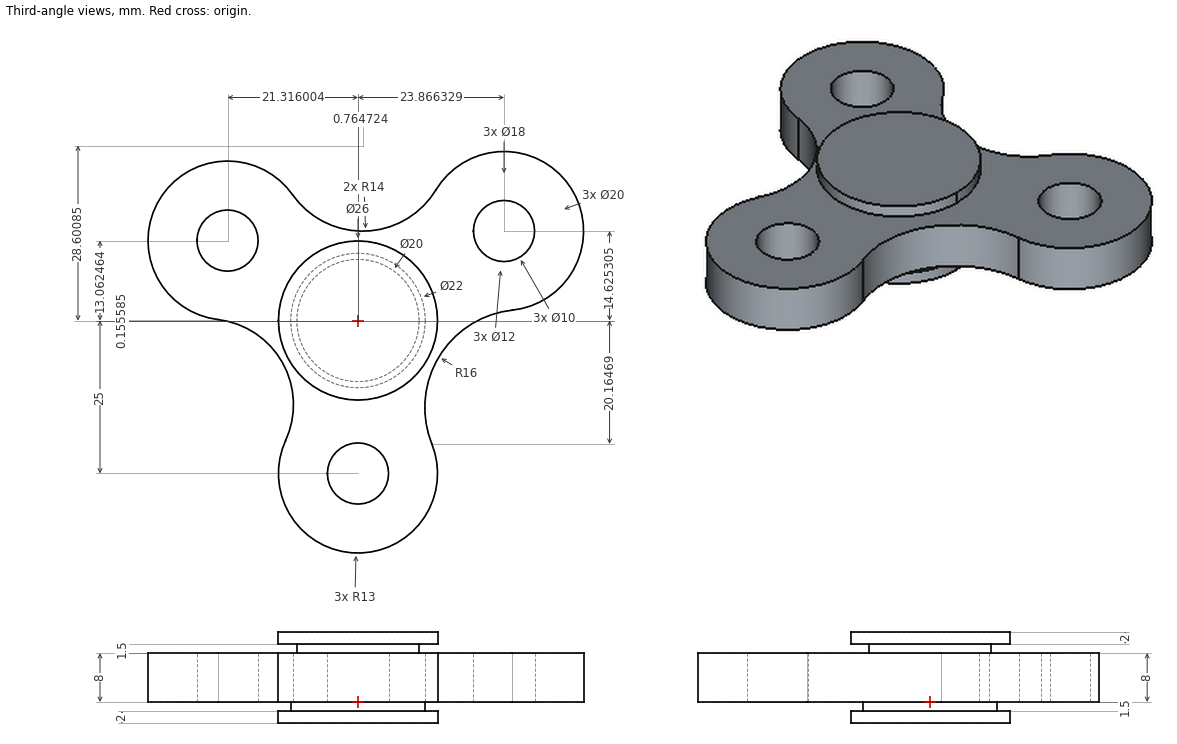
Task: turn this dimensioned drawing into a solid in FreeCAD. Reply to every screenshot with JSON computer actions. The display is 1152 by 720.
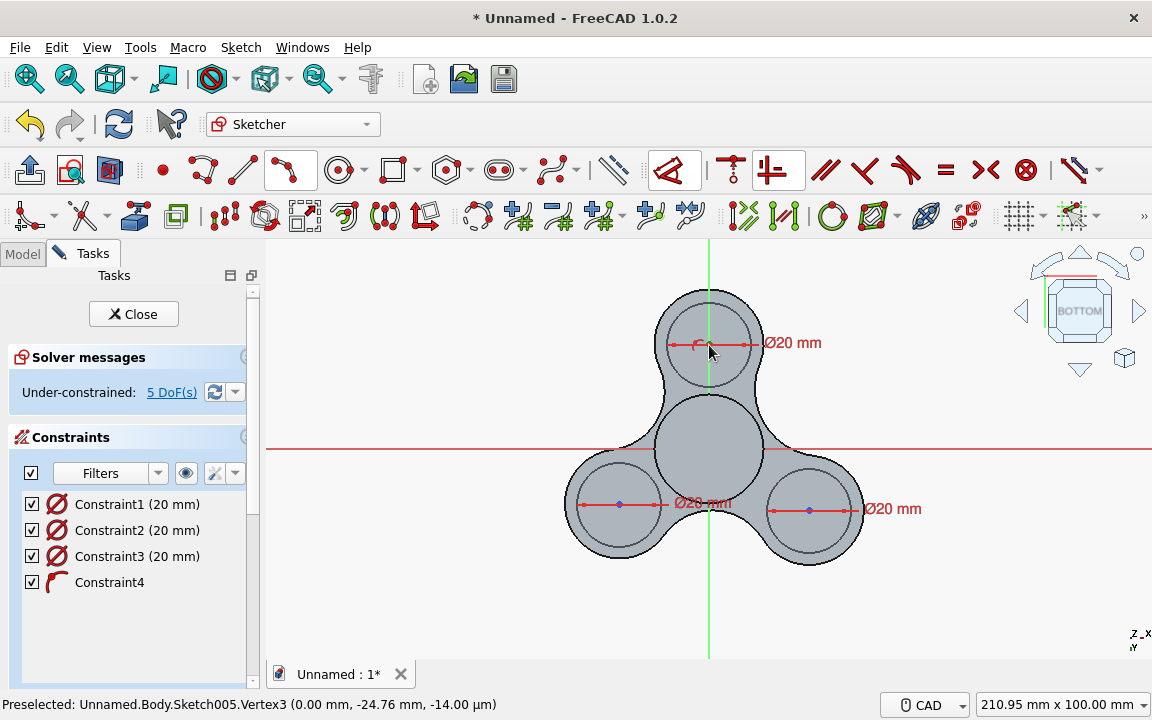
{"action": "left_click", "coordinate": [696, 170]}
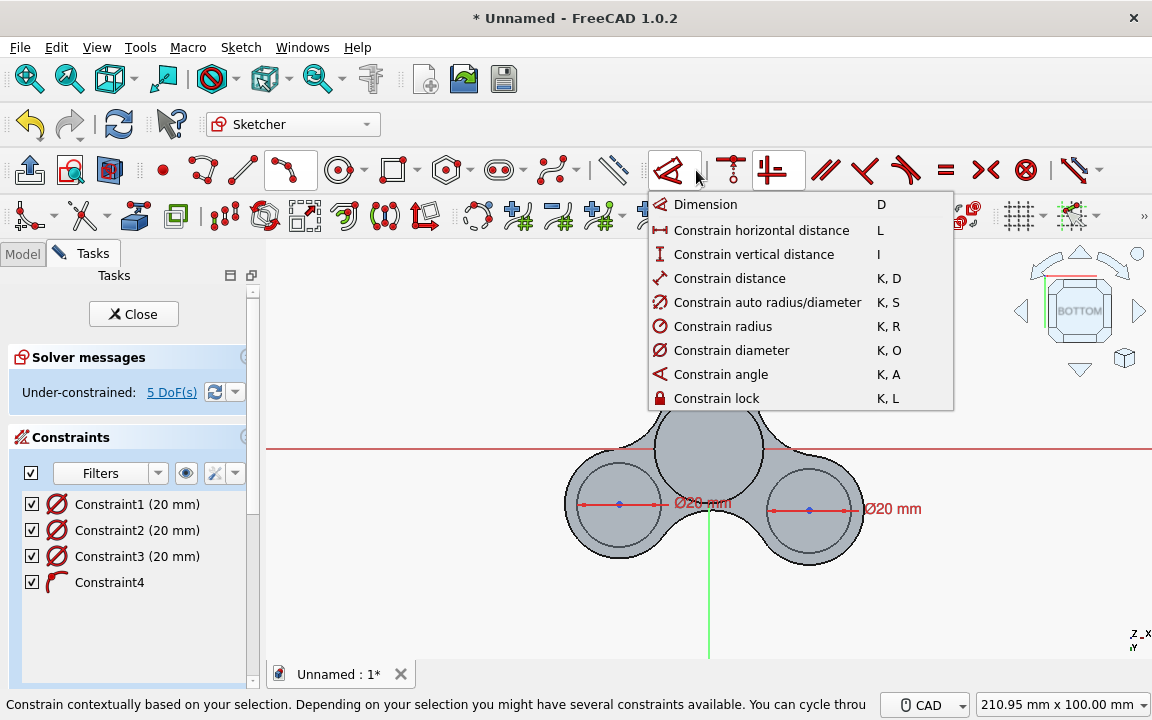
{"action": "left_click", "coordinate": [801, 254]}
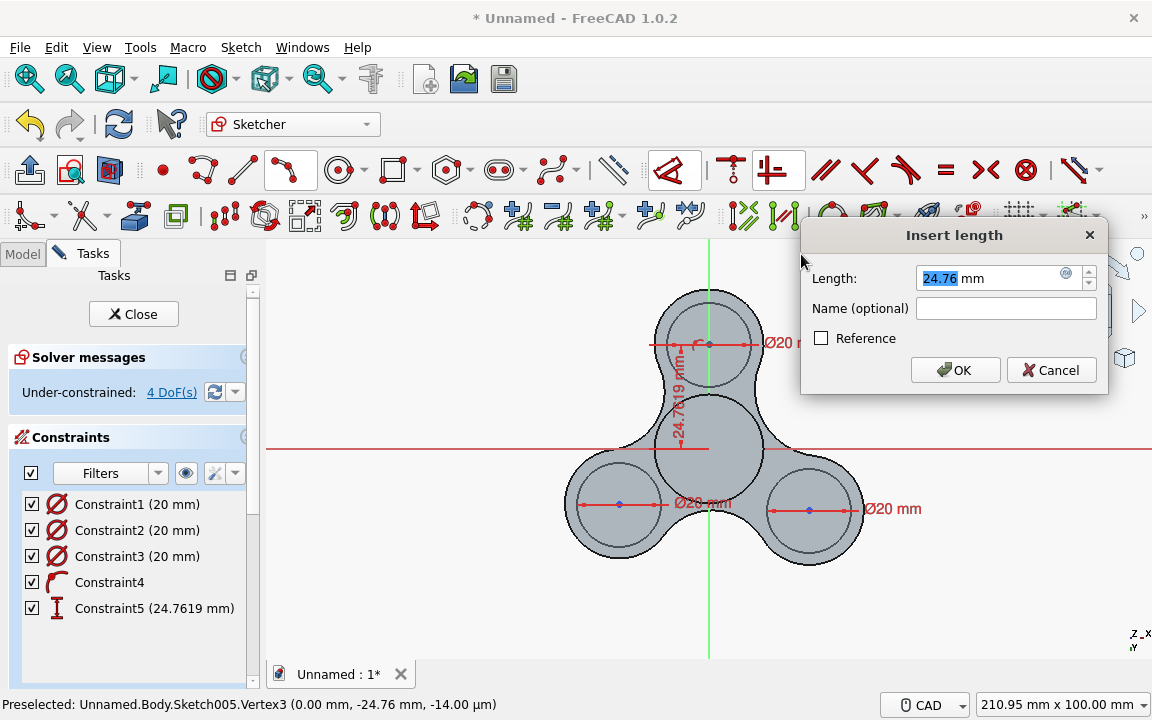
{"action": "type", "text": "25"}
{"action": "key", "text": "Return"}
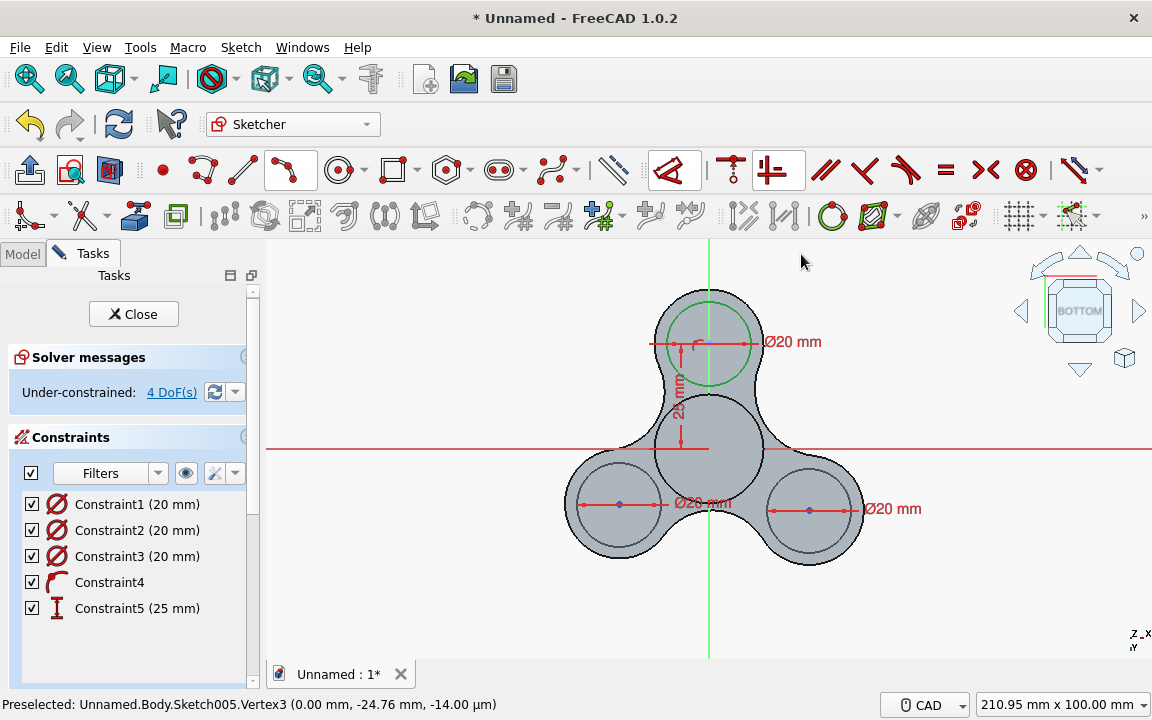
{"action": "left_click", "coordinate": [809, 511]}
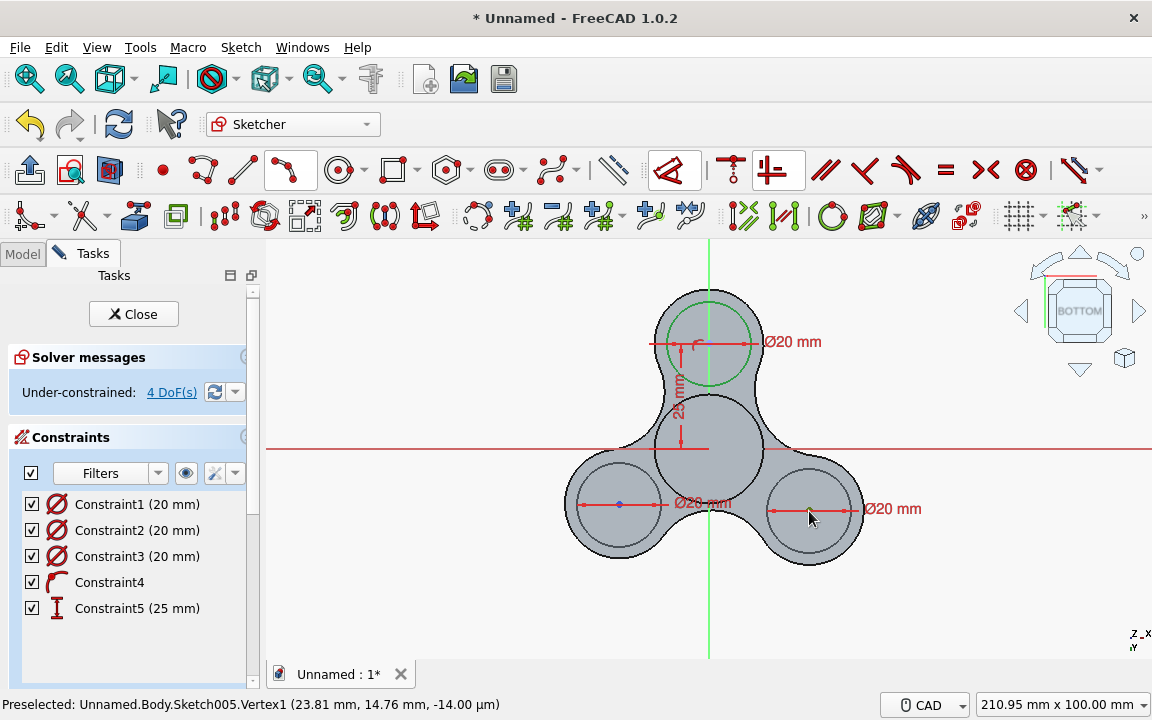
{"action": "key", "text": "l"}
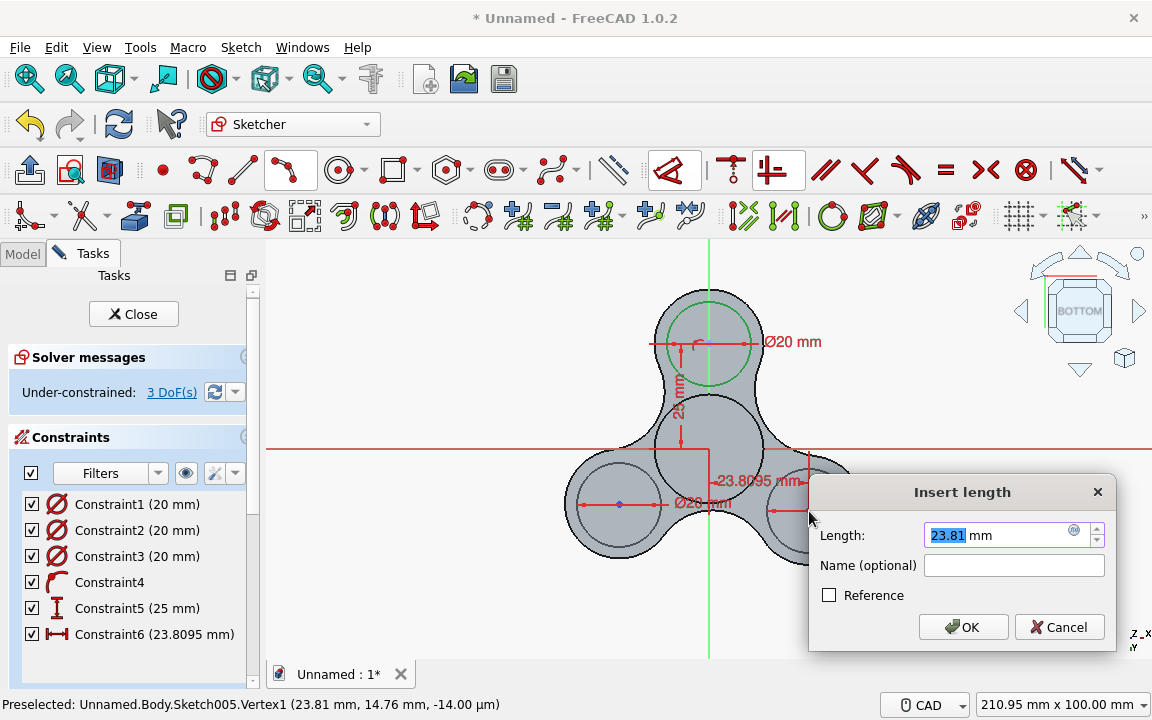
{"action": "type", "text": "23.866329"}
{"action": "key", "text": "Return"}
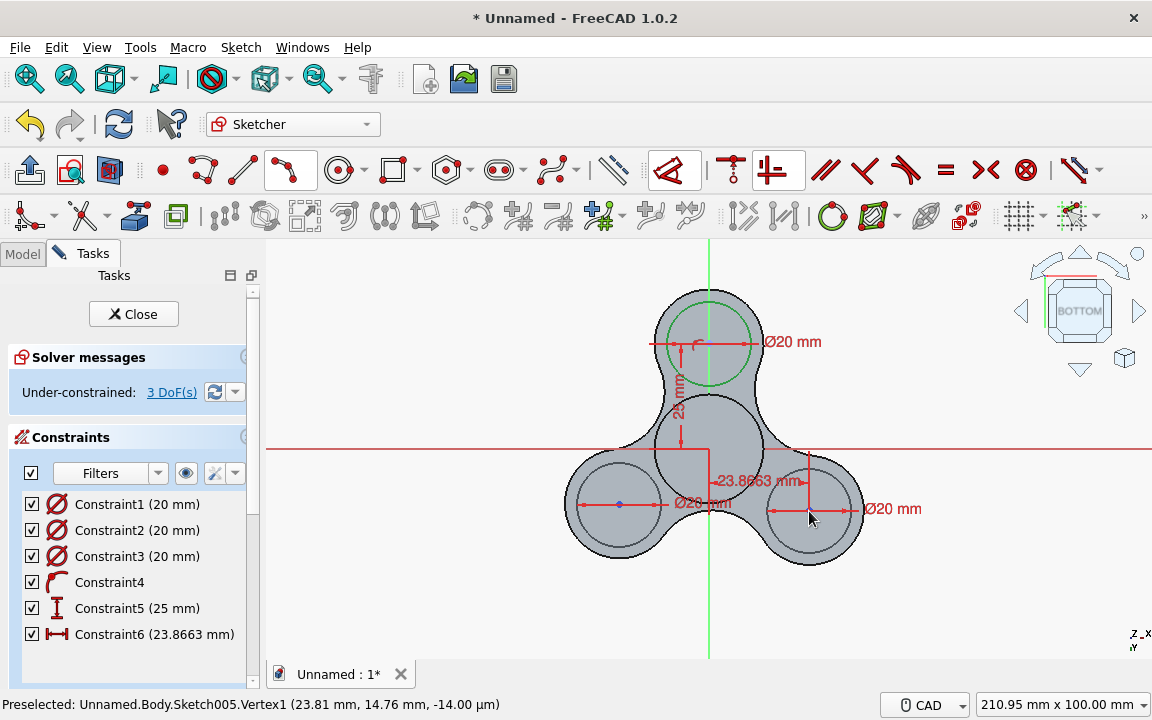
{"action": "left_click", "coordinate": [809, 511]}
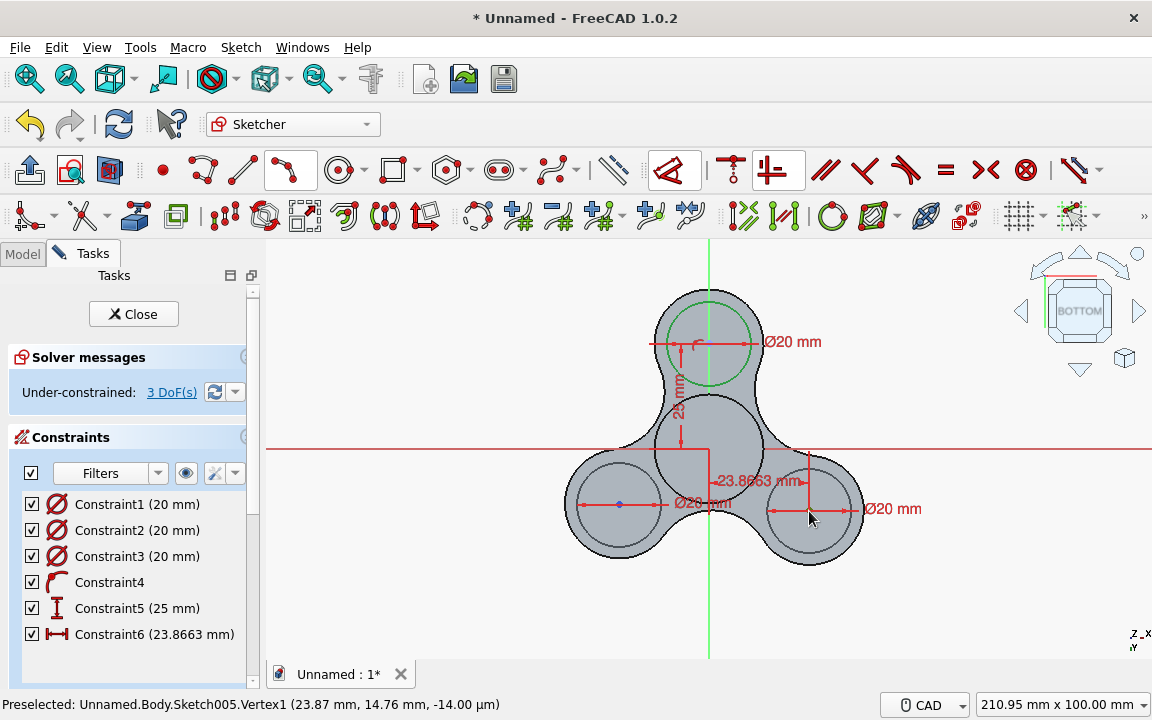
{"action": "key", "text": "i"}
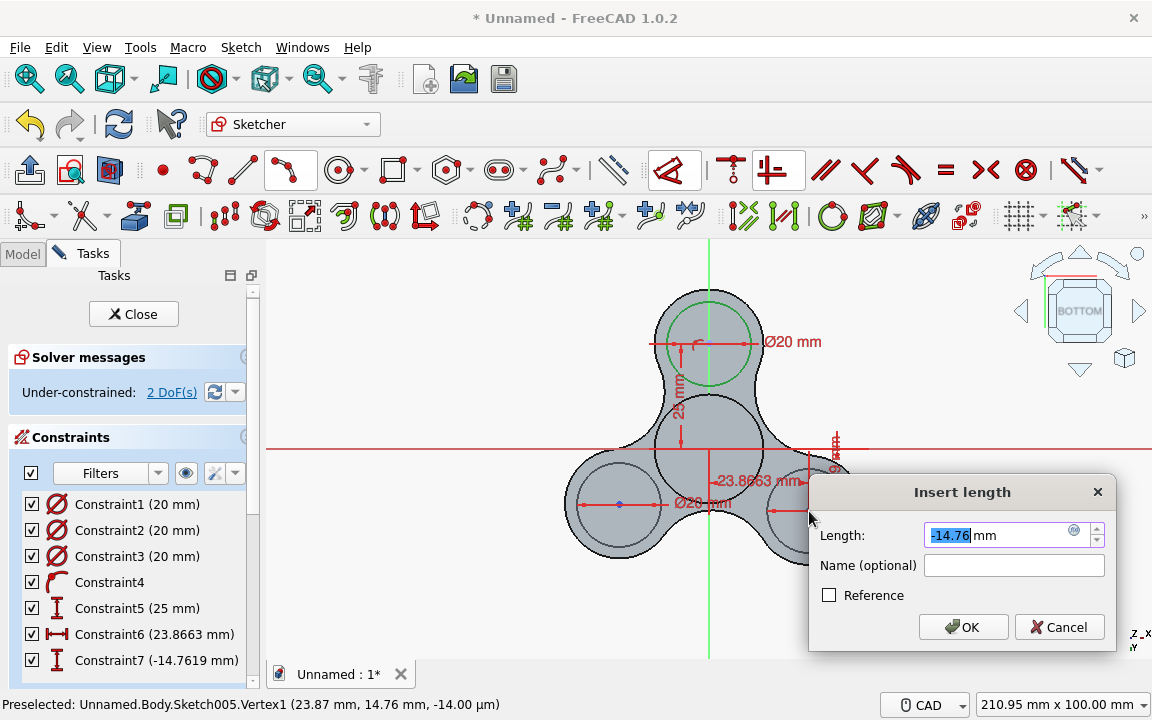
{"action": "type", "text": "-14.625305"}
{"action": "key", "text": "Return"}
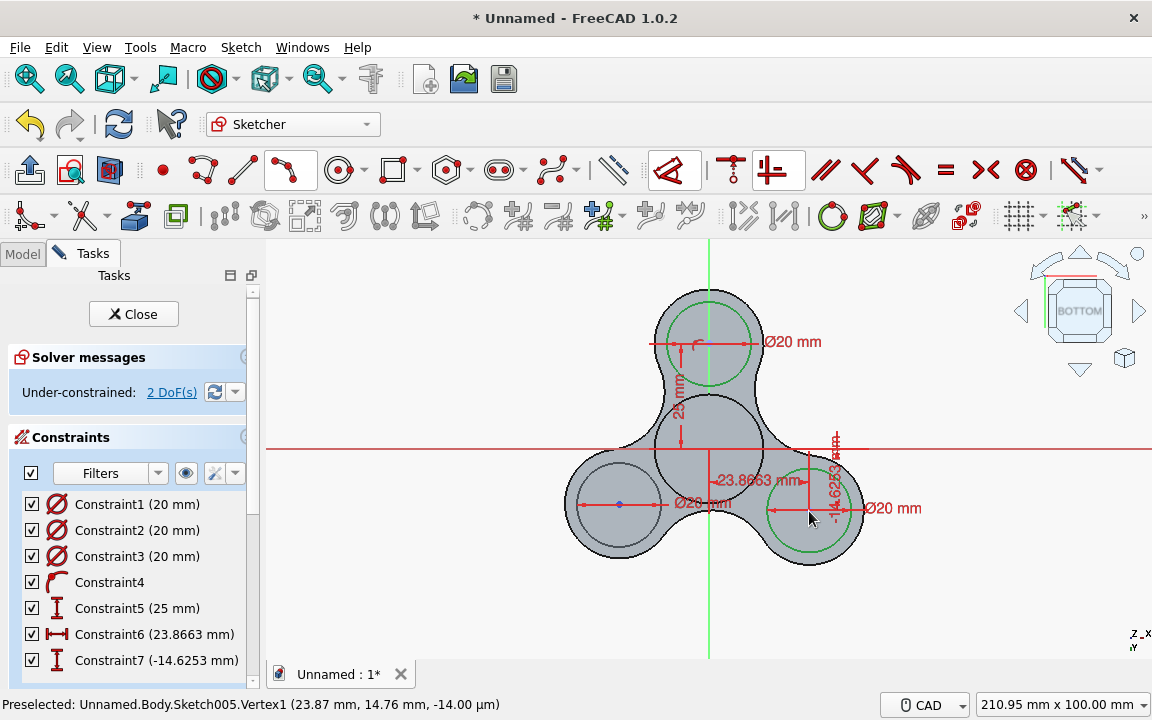
{"action": "left_click", "coordinate": [619, 505]}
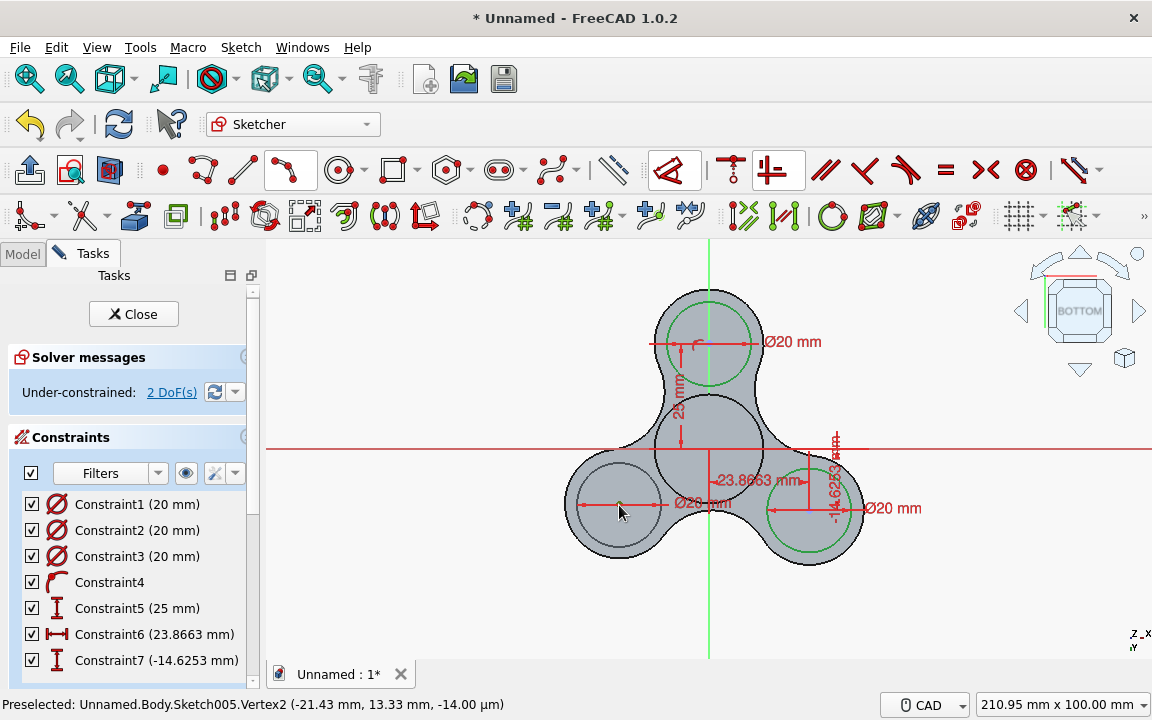
{"action": "key", "text": "l"}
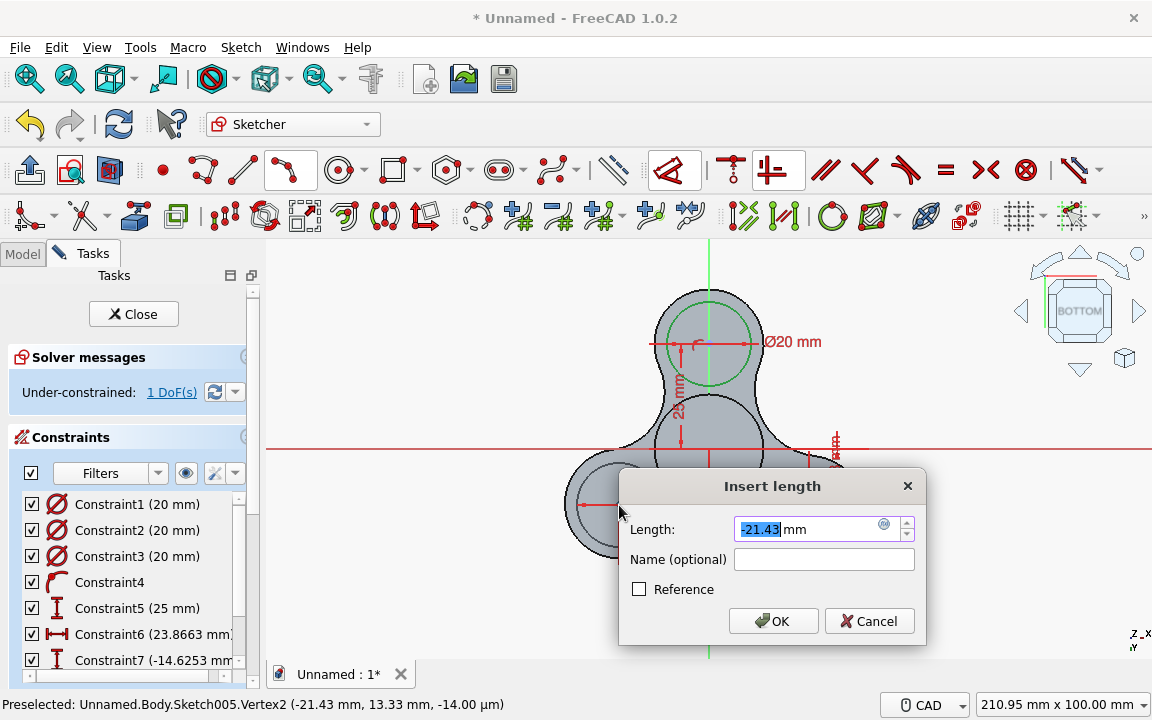
{"action": "type", "text": "-21.316004"}
{"action": "key", "text": "Return"}